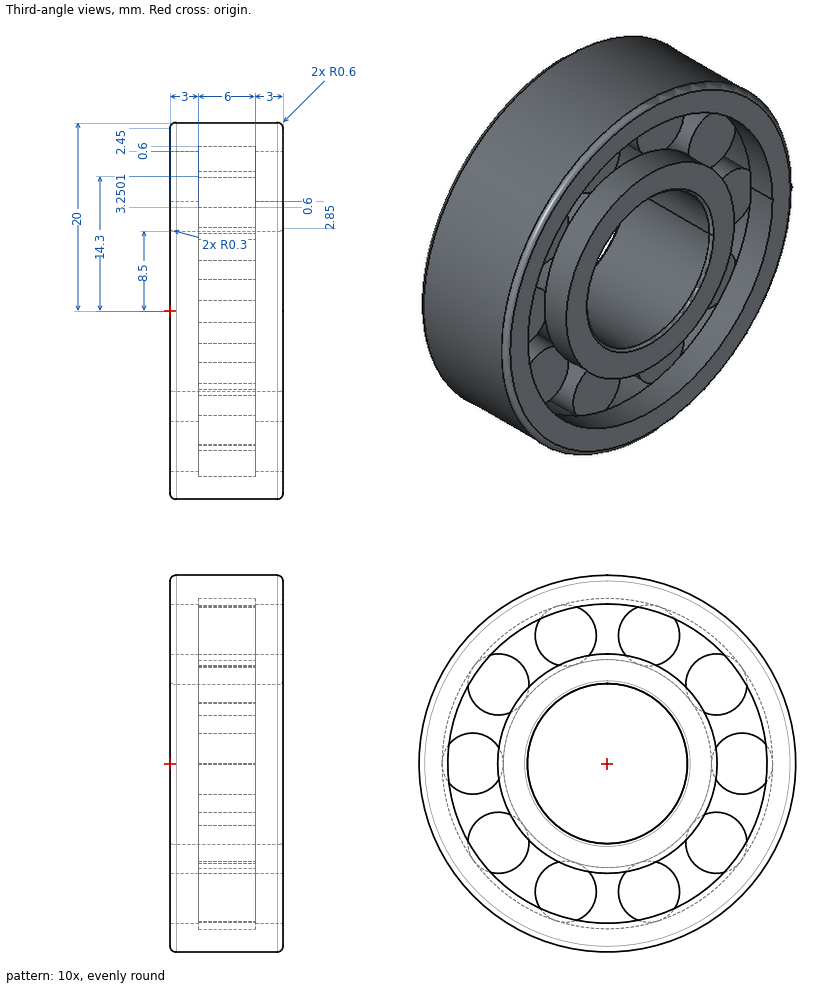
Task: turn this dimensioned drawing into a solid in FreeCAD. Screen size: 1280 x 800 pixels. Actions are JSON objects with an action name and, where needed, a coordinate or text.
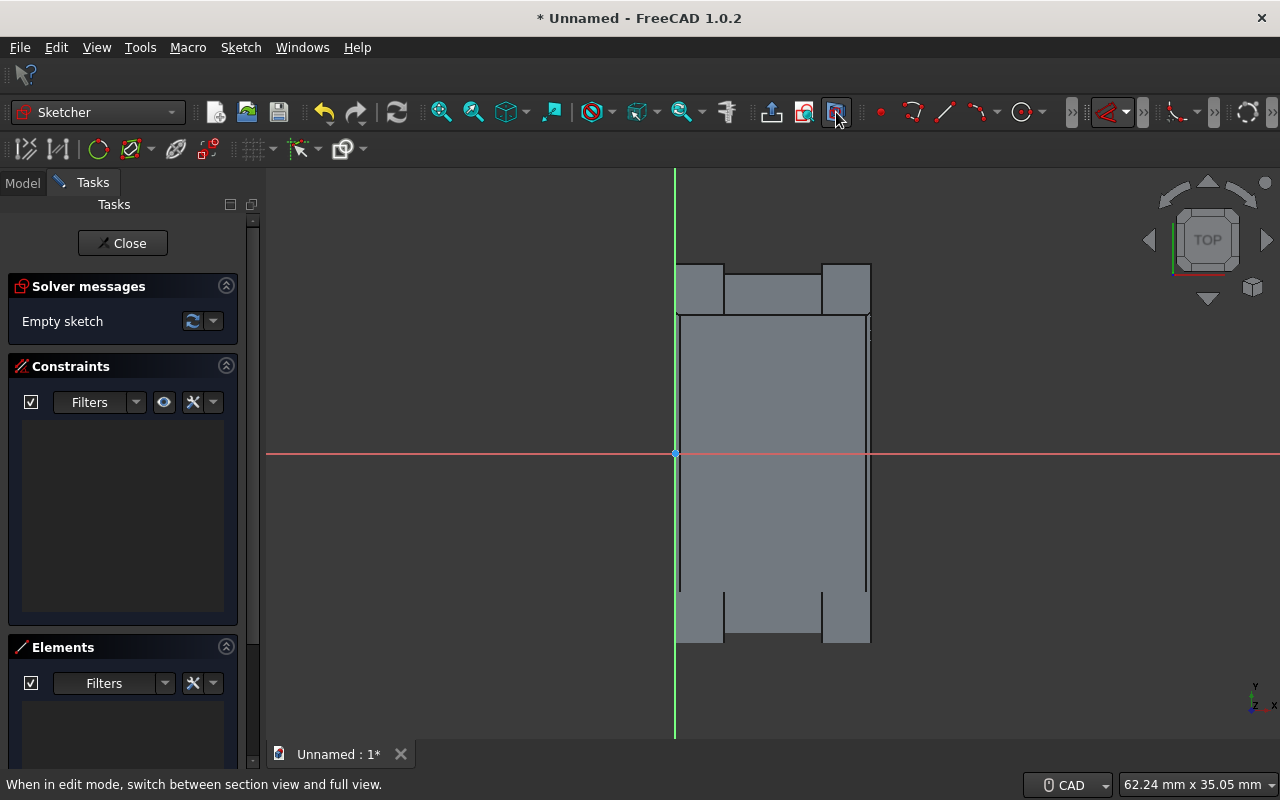
{"action": "scroll", "coordinate": [897, 196], "scroll_direction": "up", "scroll_amount": 2}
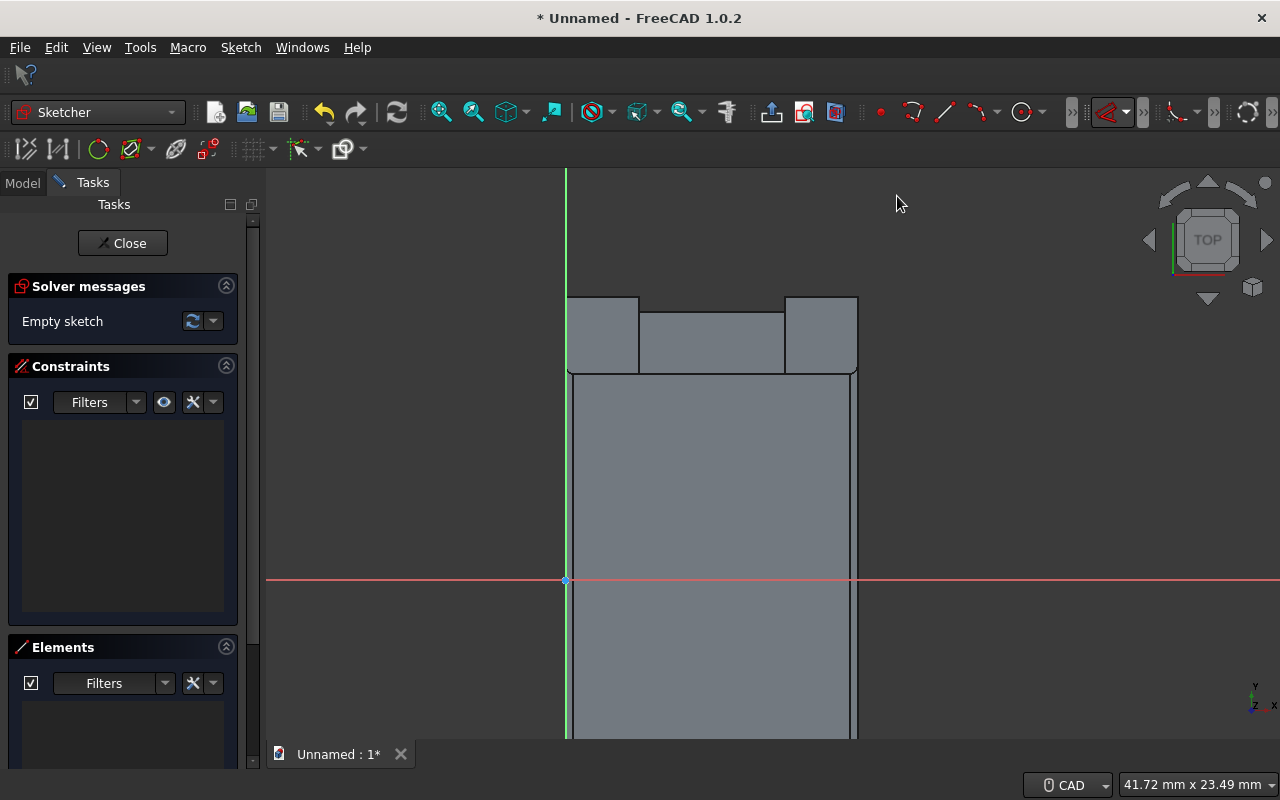
{"action": "key", "text": "g r"}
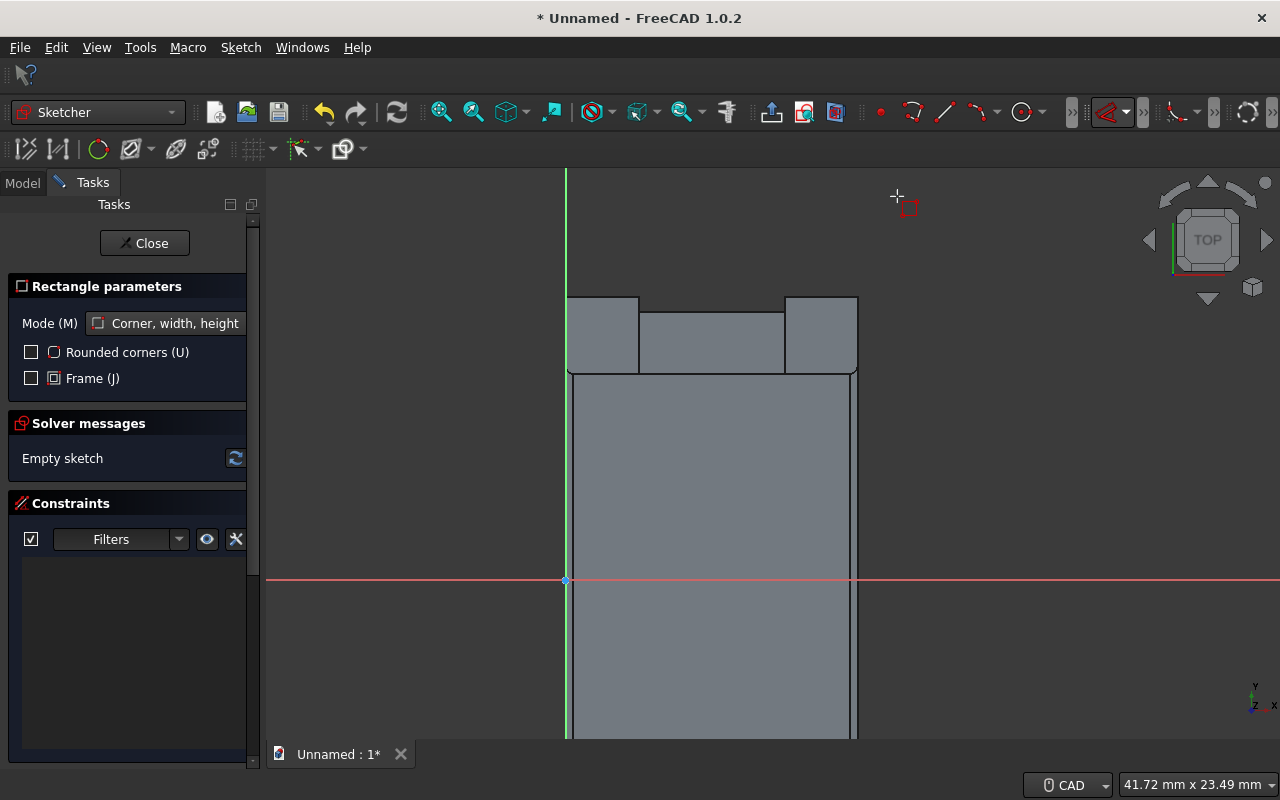
{"action": "left_click", "coordinate": [639, 233]}
{"action": "left_click", "coordinate": [785, 312]}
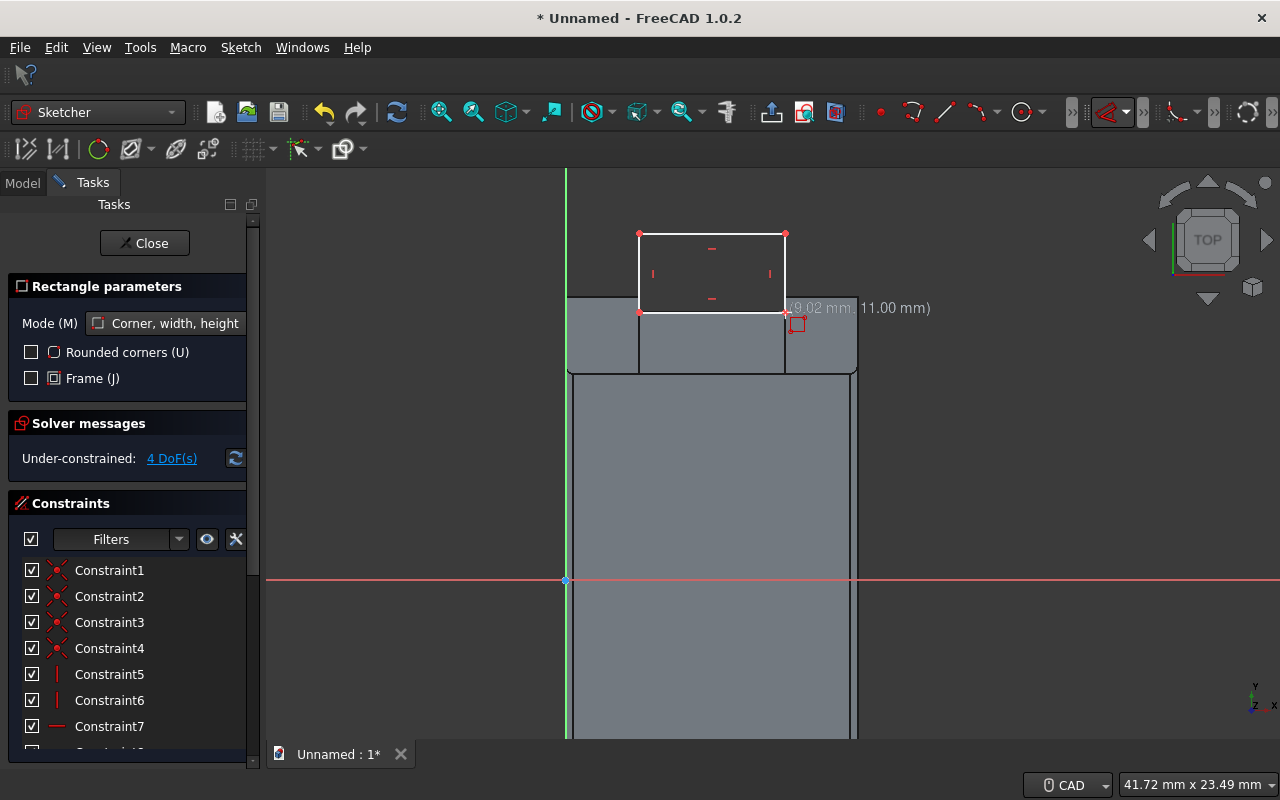
{"action": "left_click", "coordinate": [946, 112]}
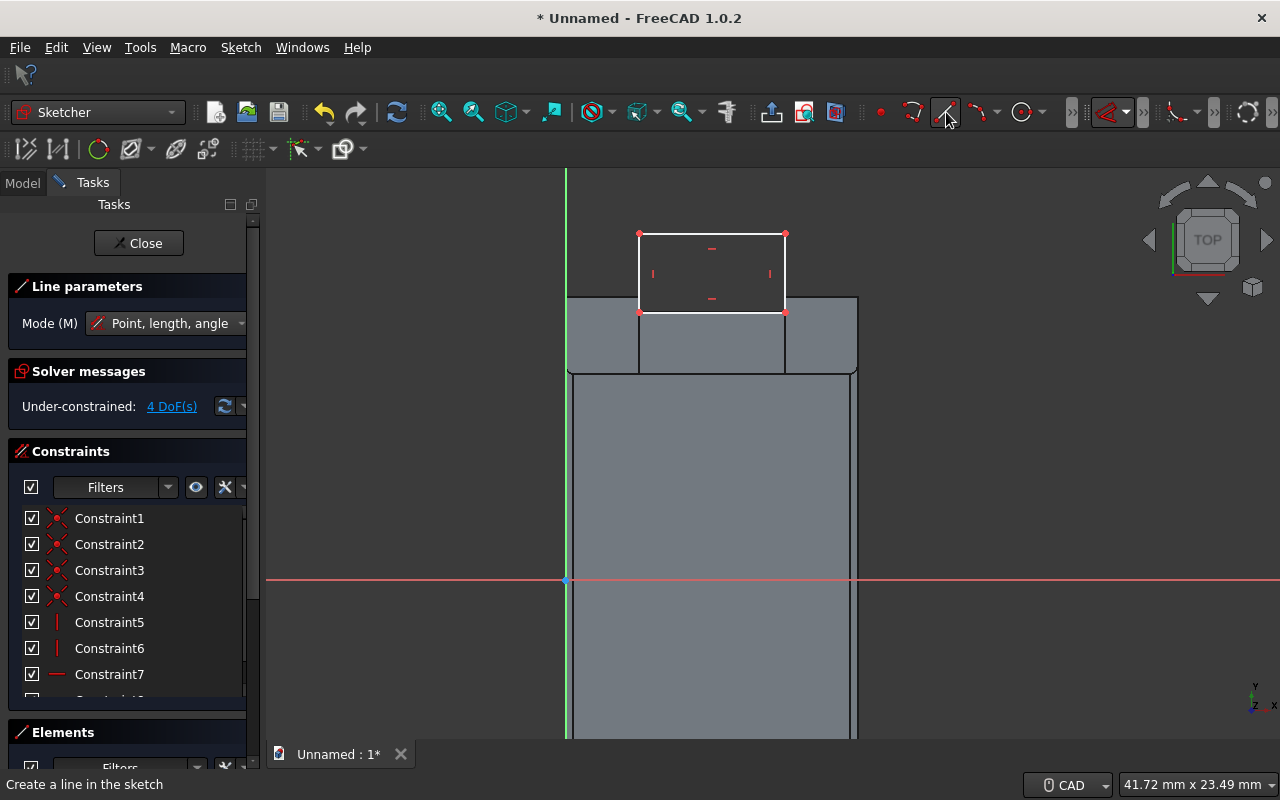
{"action": "left_click", "coordinate": [799, 233]}
{"action": "left_click", "coordinate": [843, 233]}
{"action": "key", "text": "Escape"}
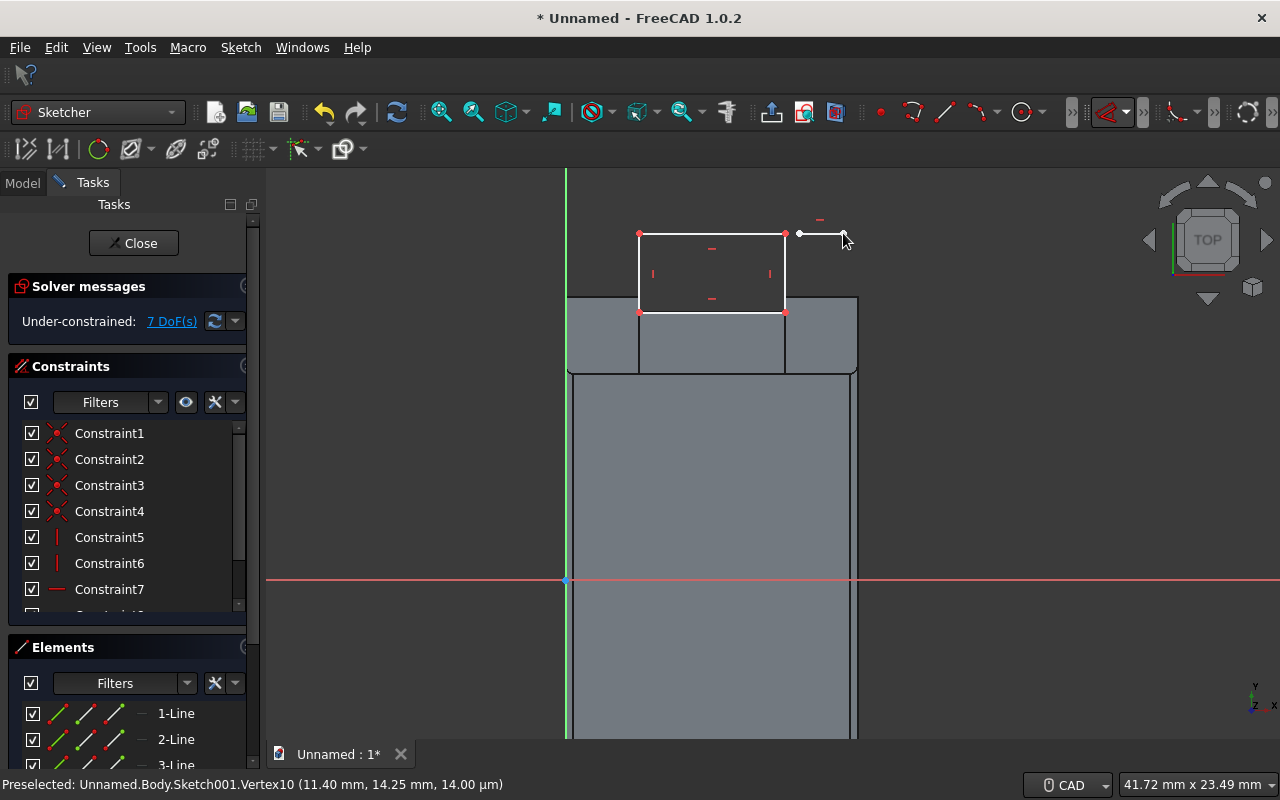
{"action": "left_click", "coordinate": [812, 234]}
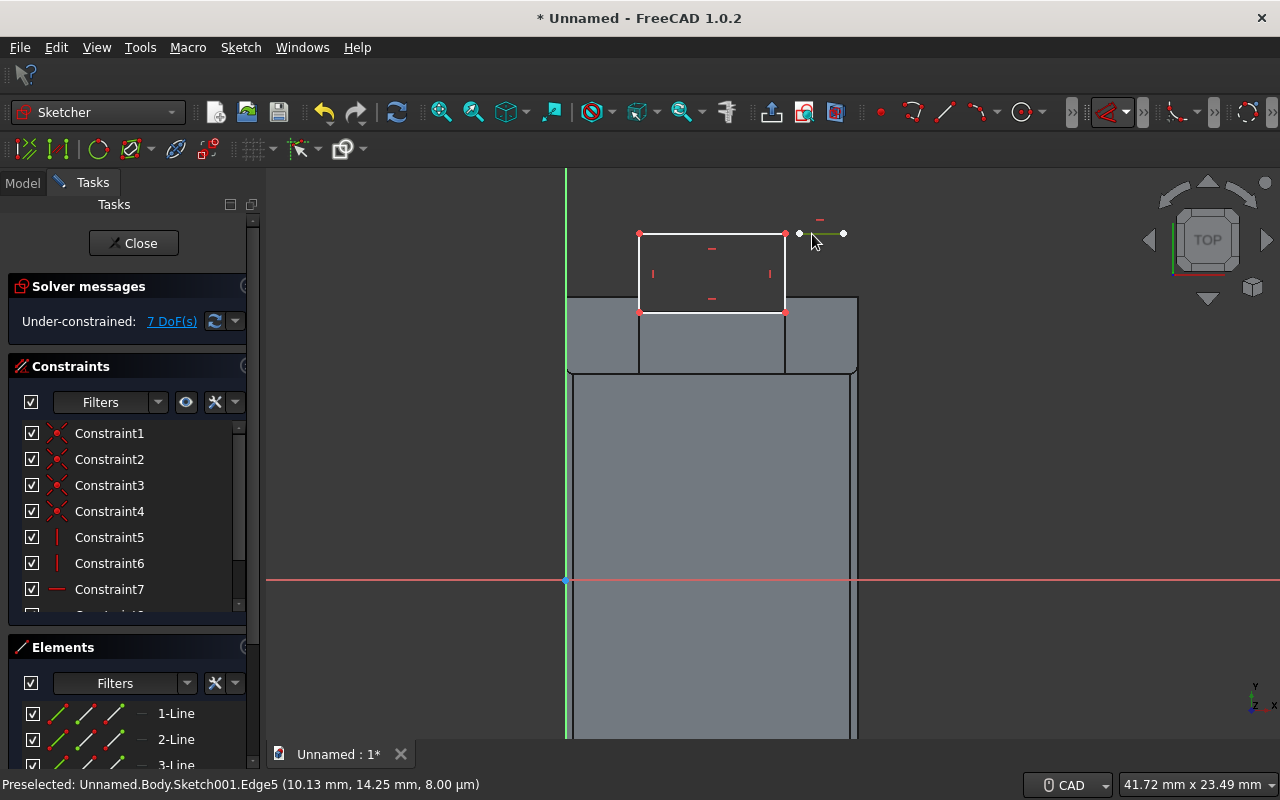
{"action": "key", "text": "g n"}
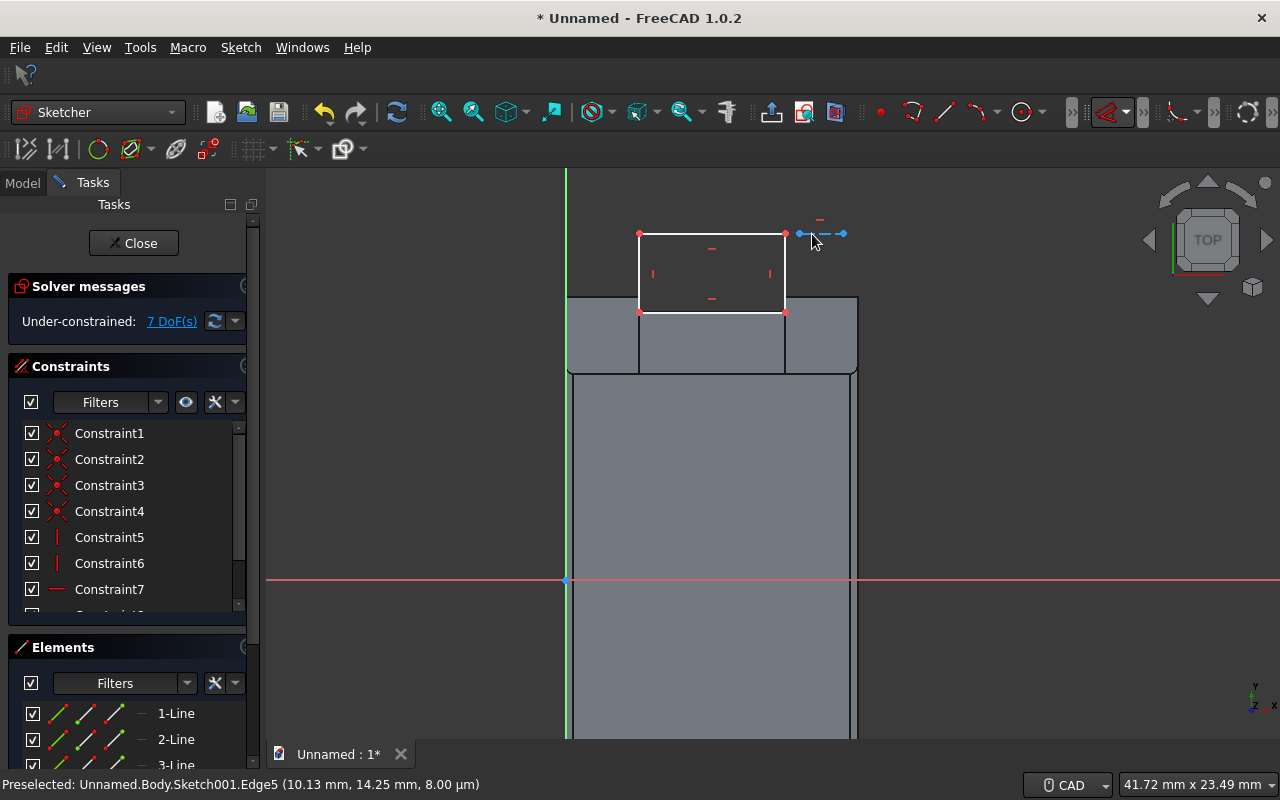
{"action": "left_click", "coordinate": [683, 313]}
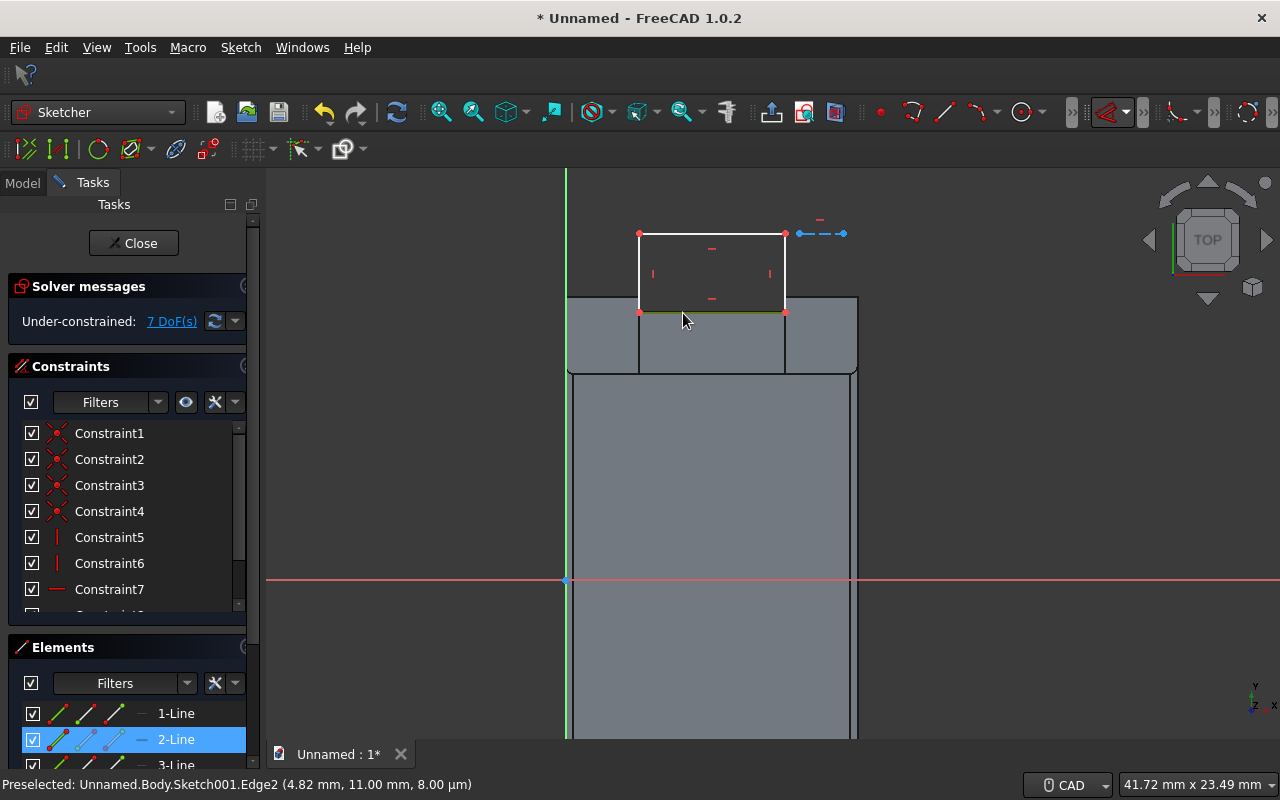
{"action": "left_click", "coordinate": [1128, 112]}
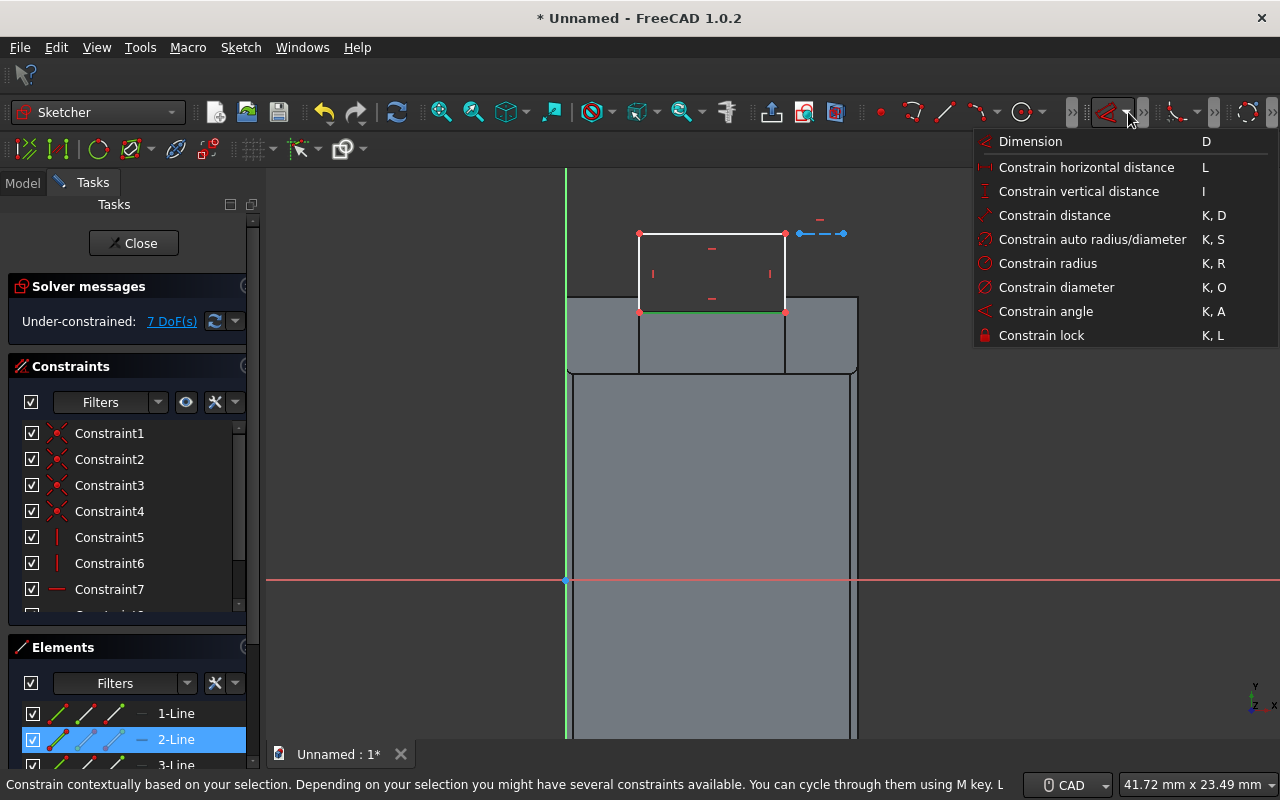
{"action": "left_click", "coordinate": [1126, 167]}